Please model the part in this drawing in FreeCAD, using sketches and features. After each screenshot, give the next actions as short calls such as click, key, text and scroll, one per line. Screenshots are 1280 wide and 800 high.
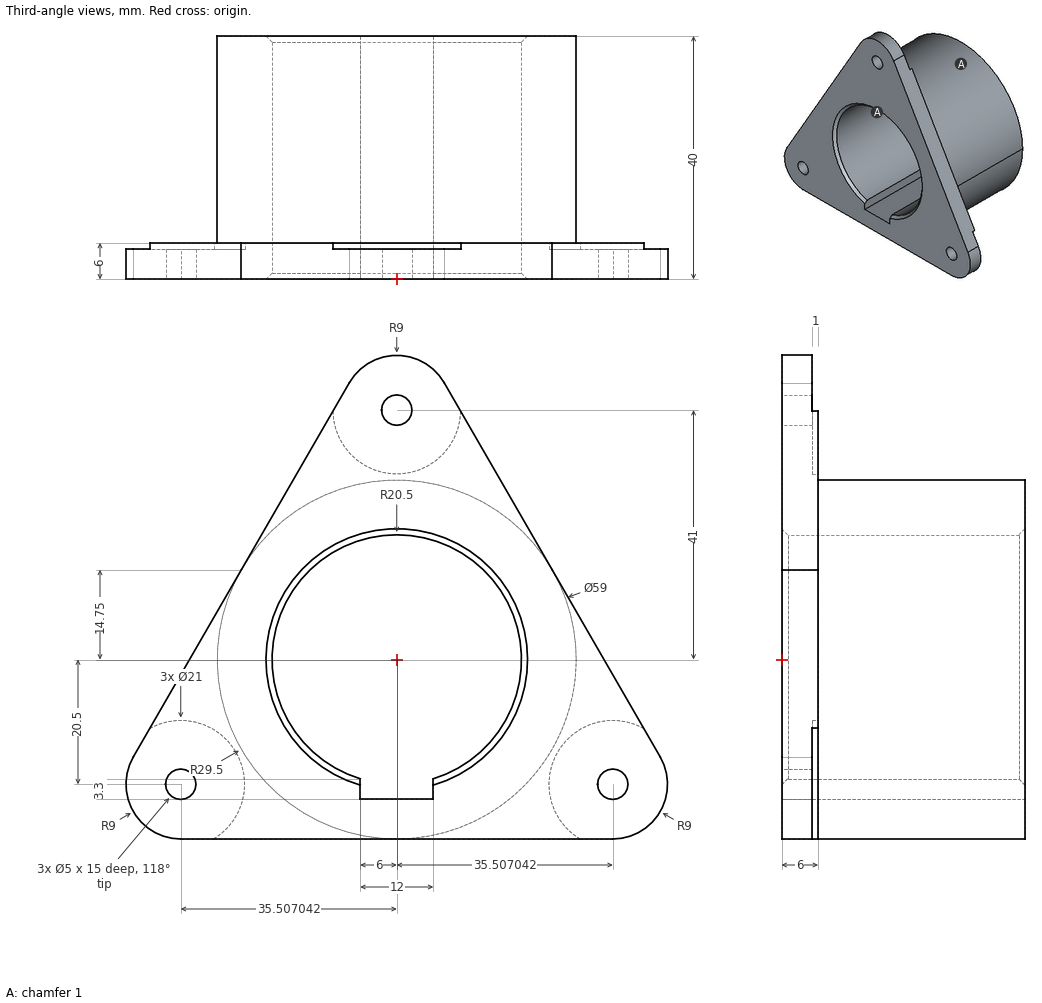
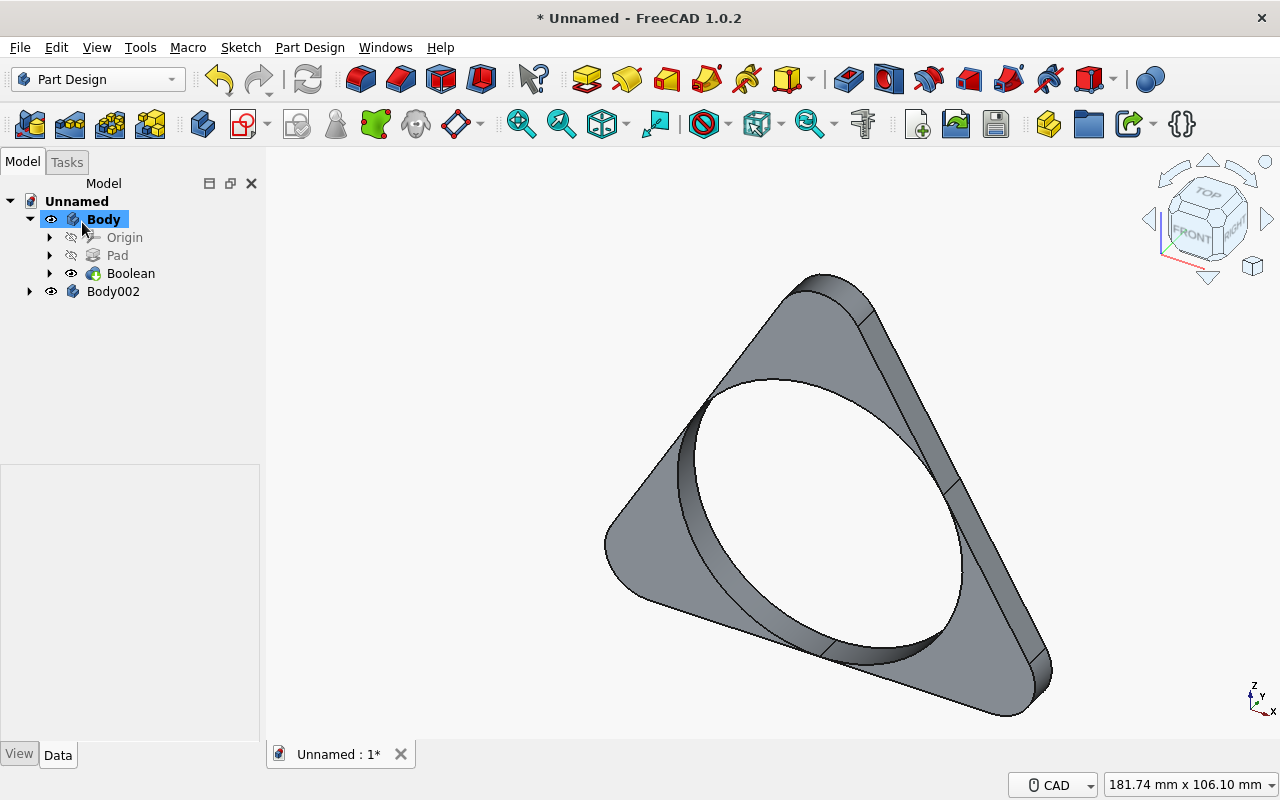
click(96, 291)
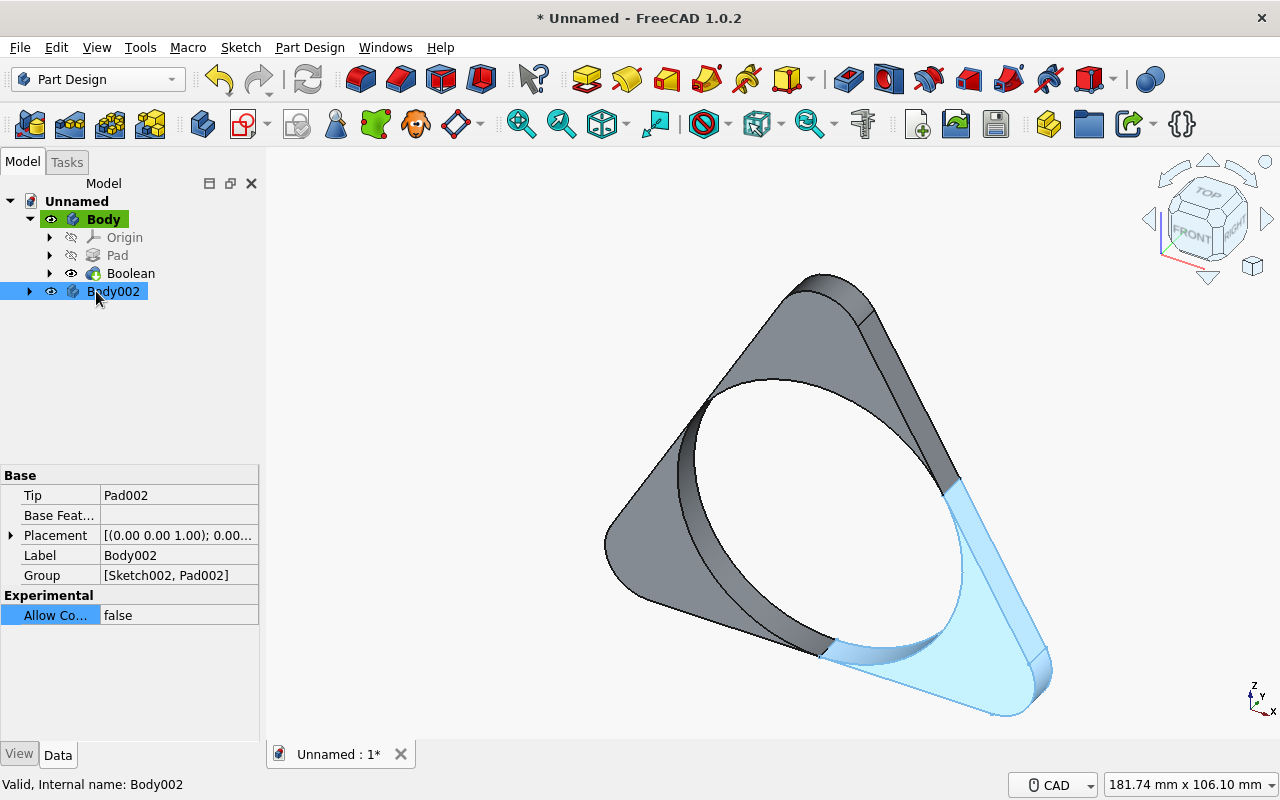
click(1152, 80)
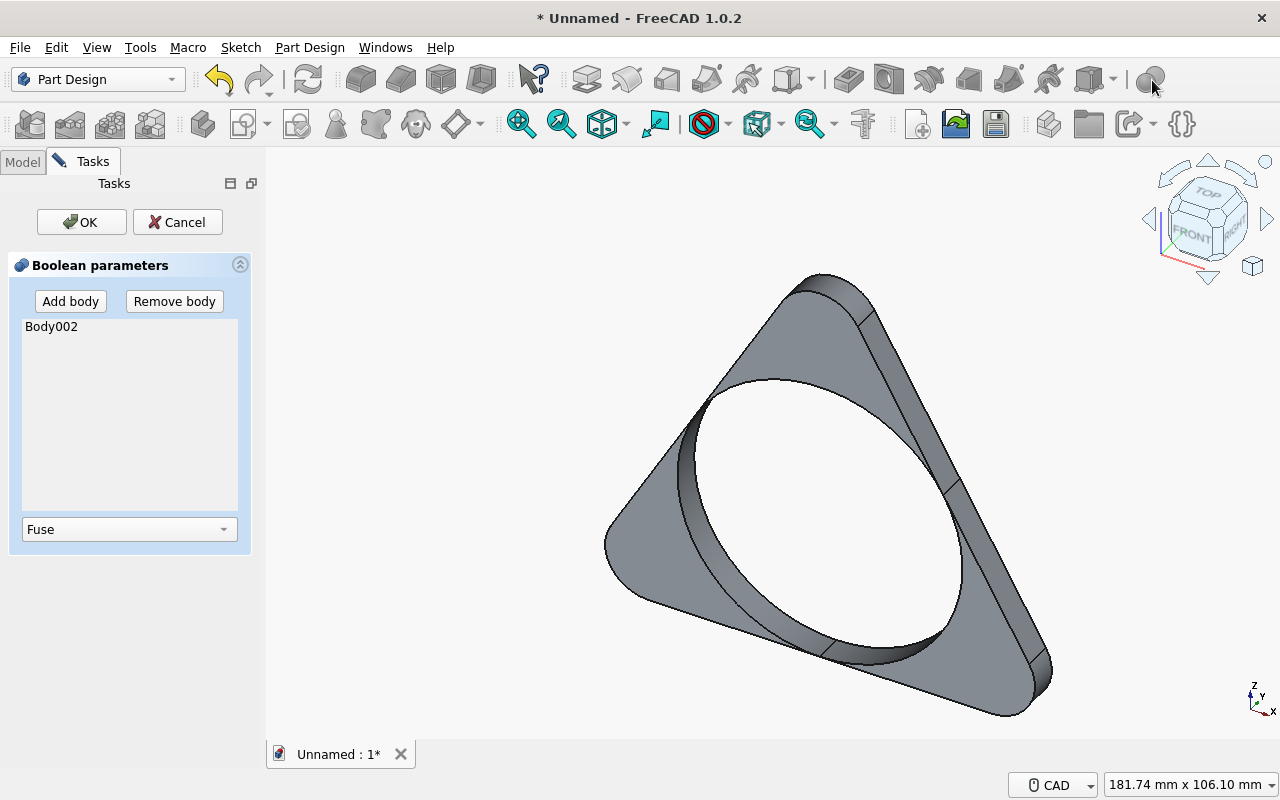
click(82, 222)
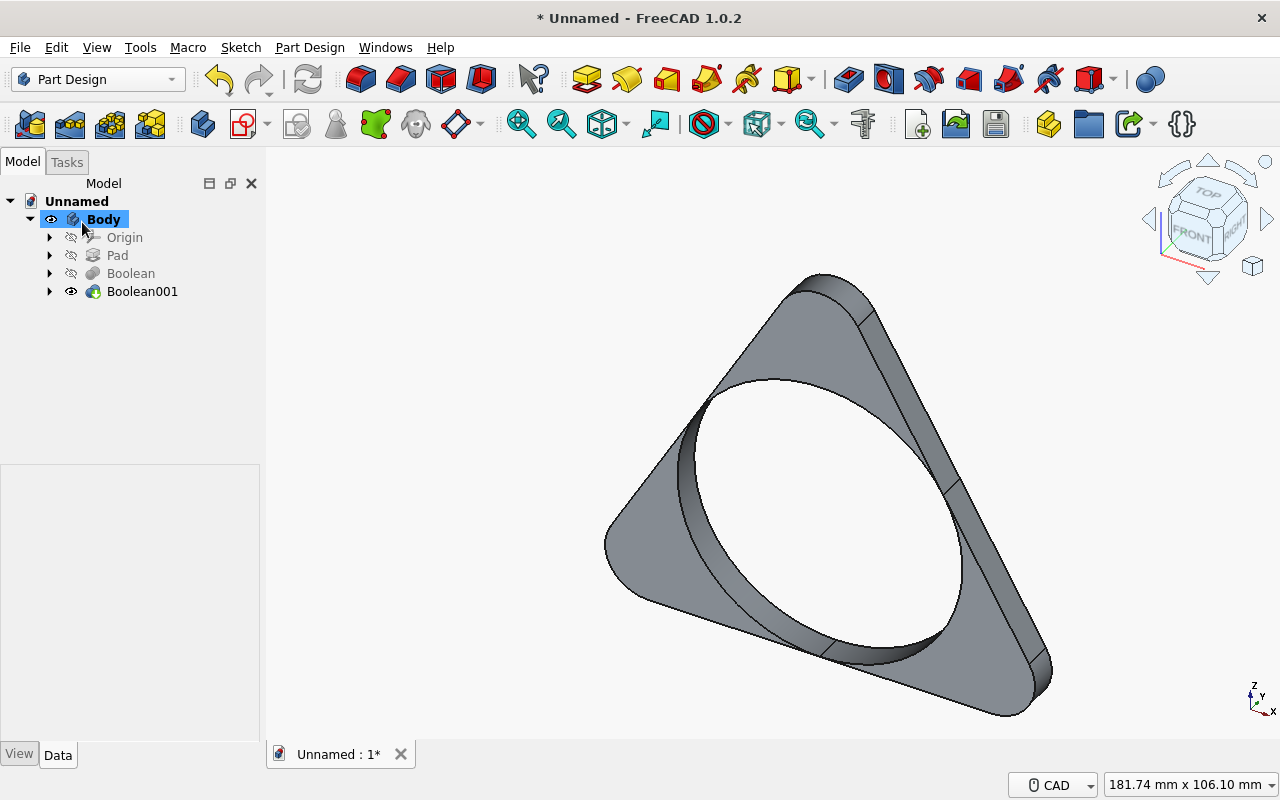
click(820, 350)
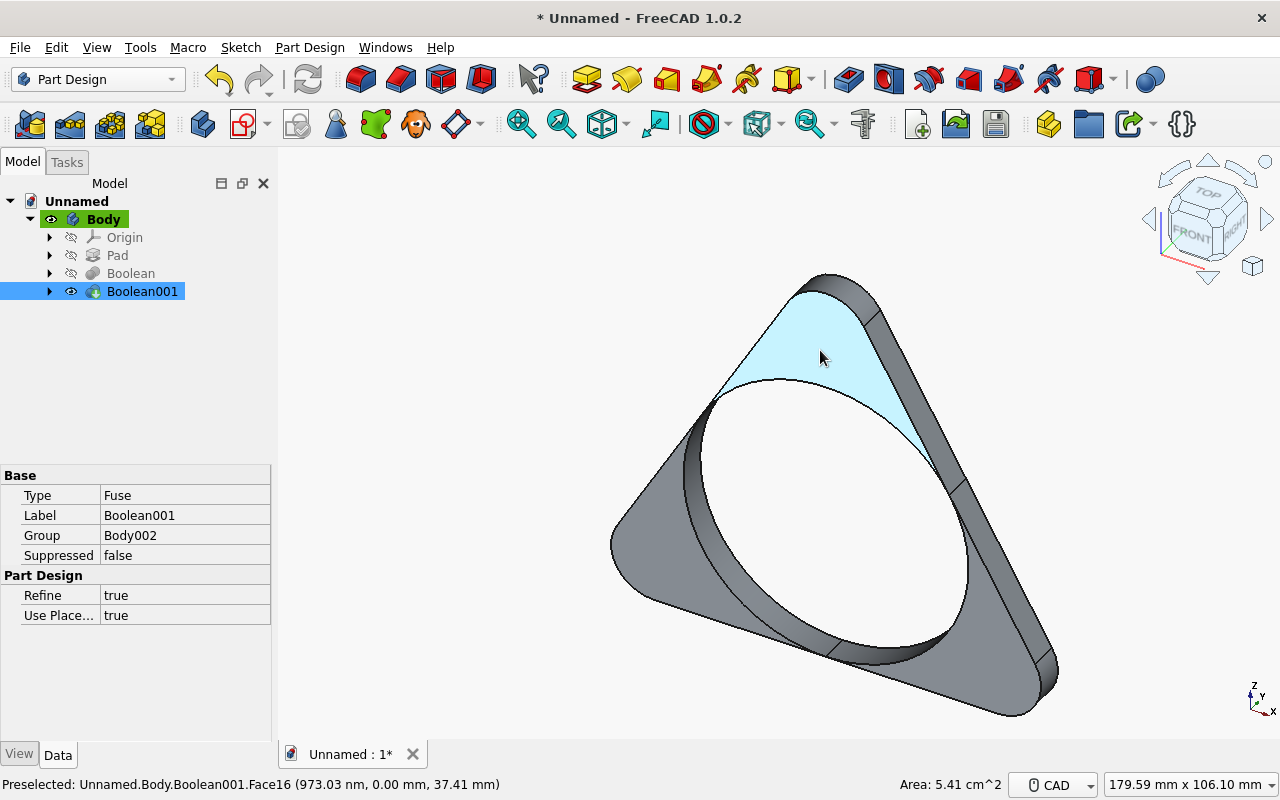
click(244, 124)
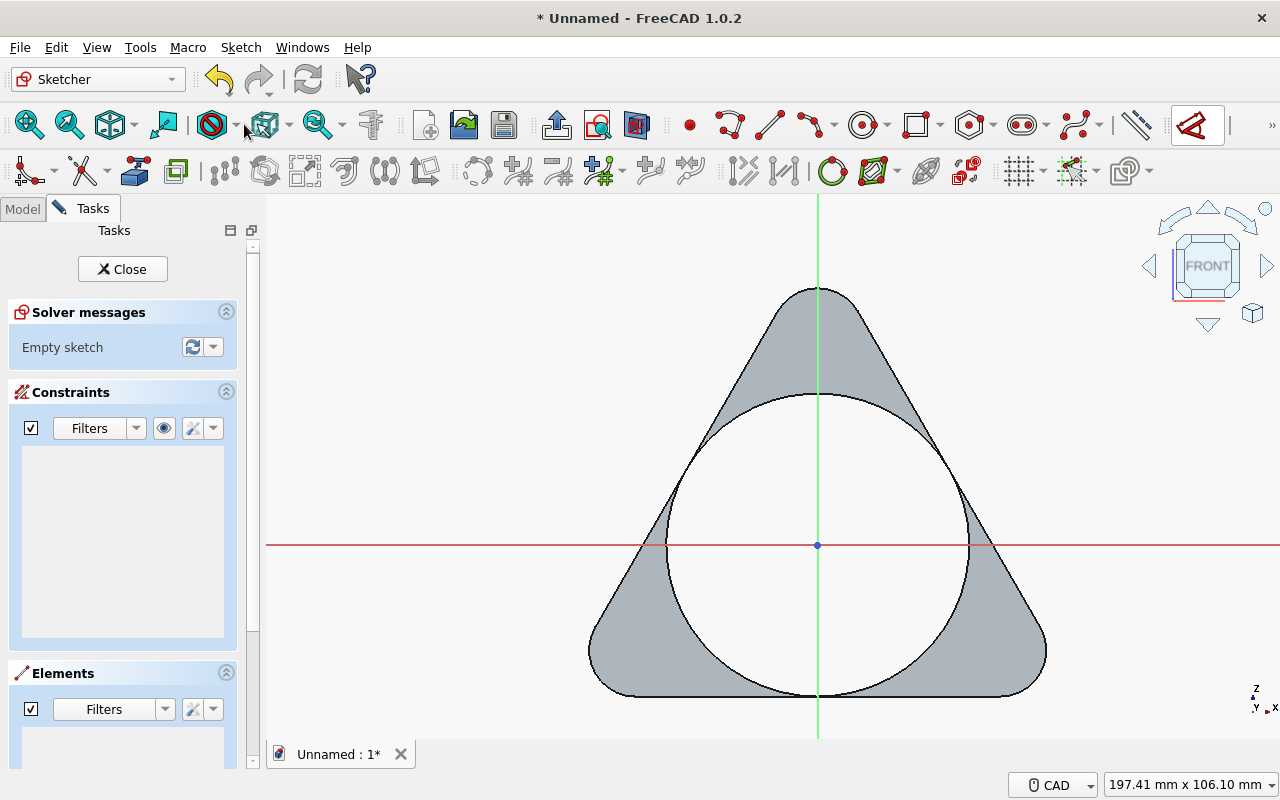
scroll(294, 222, down, 1)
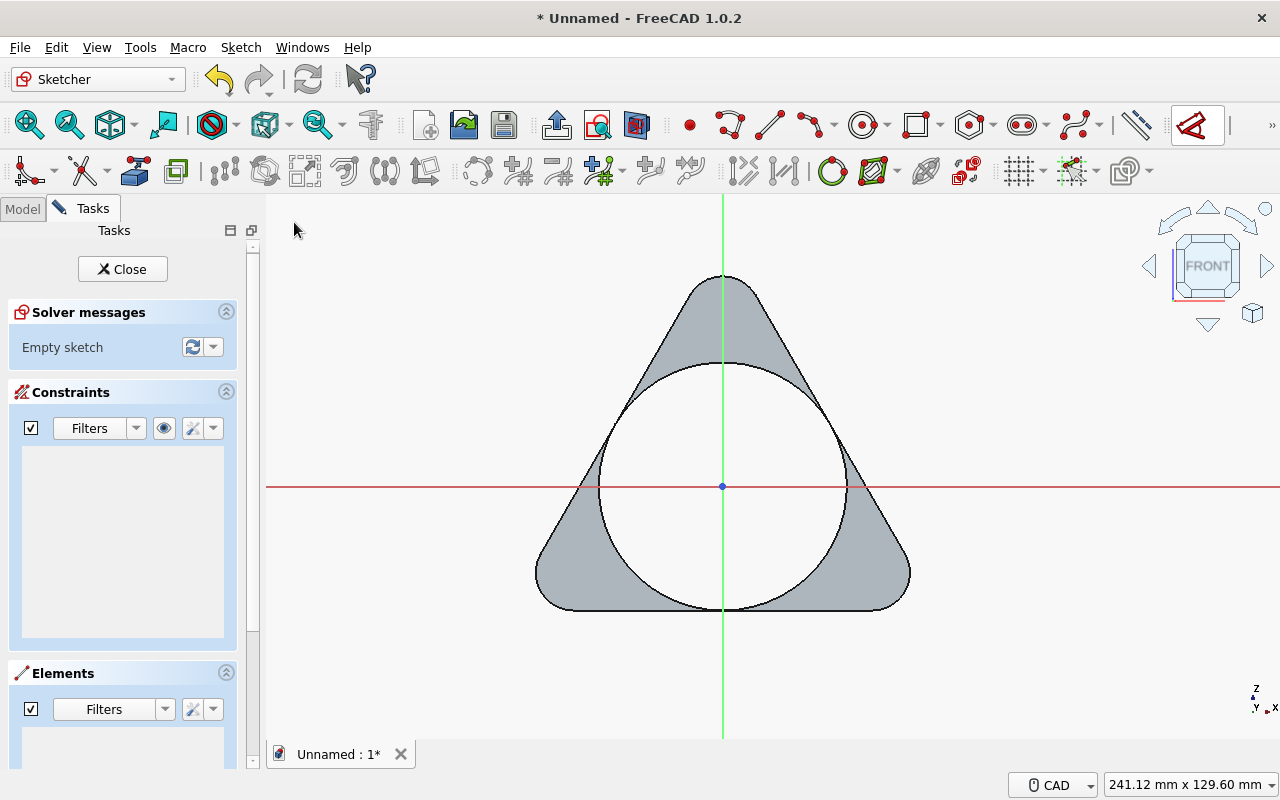
scroll(760, 527, up, 2)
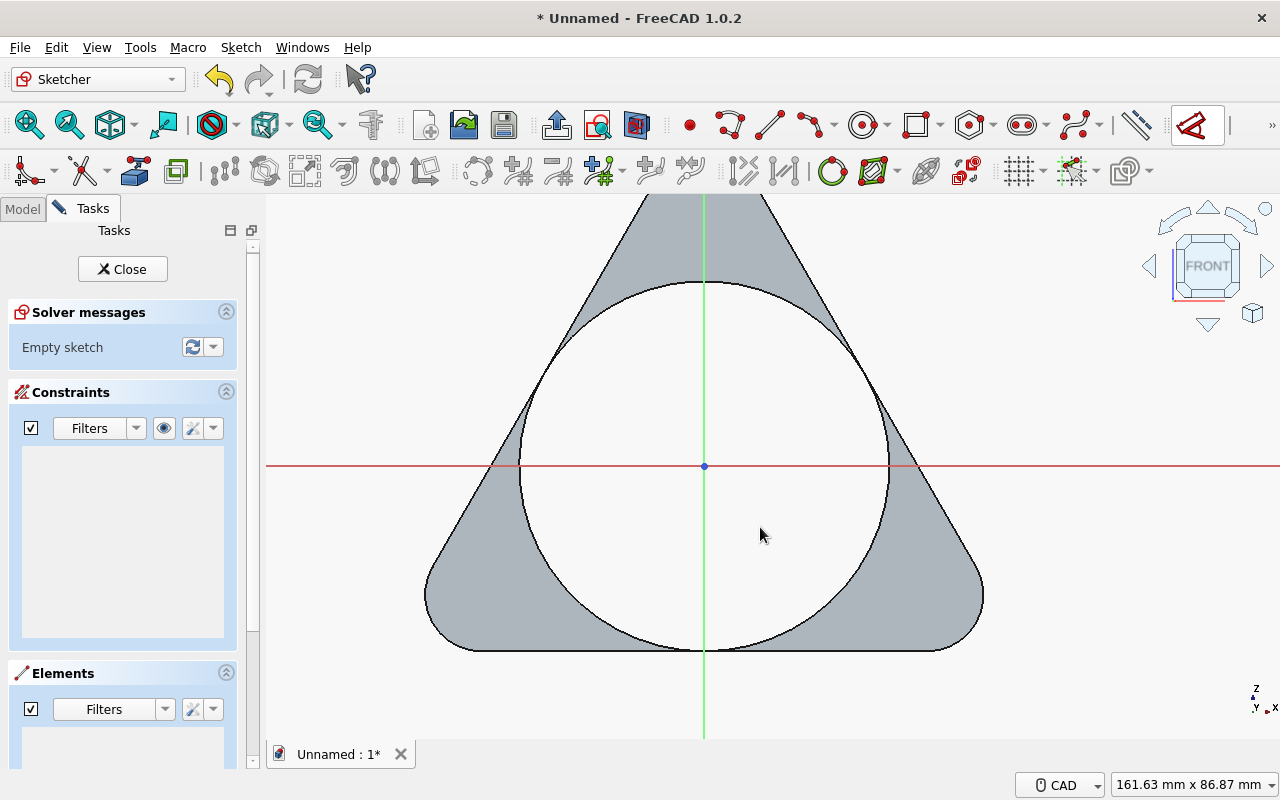
click(730, 126)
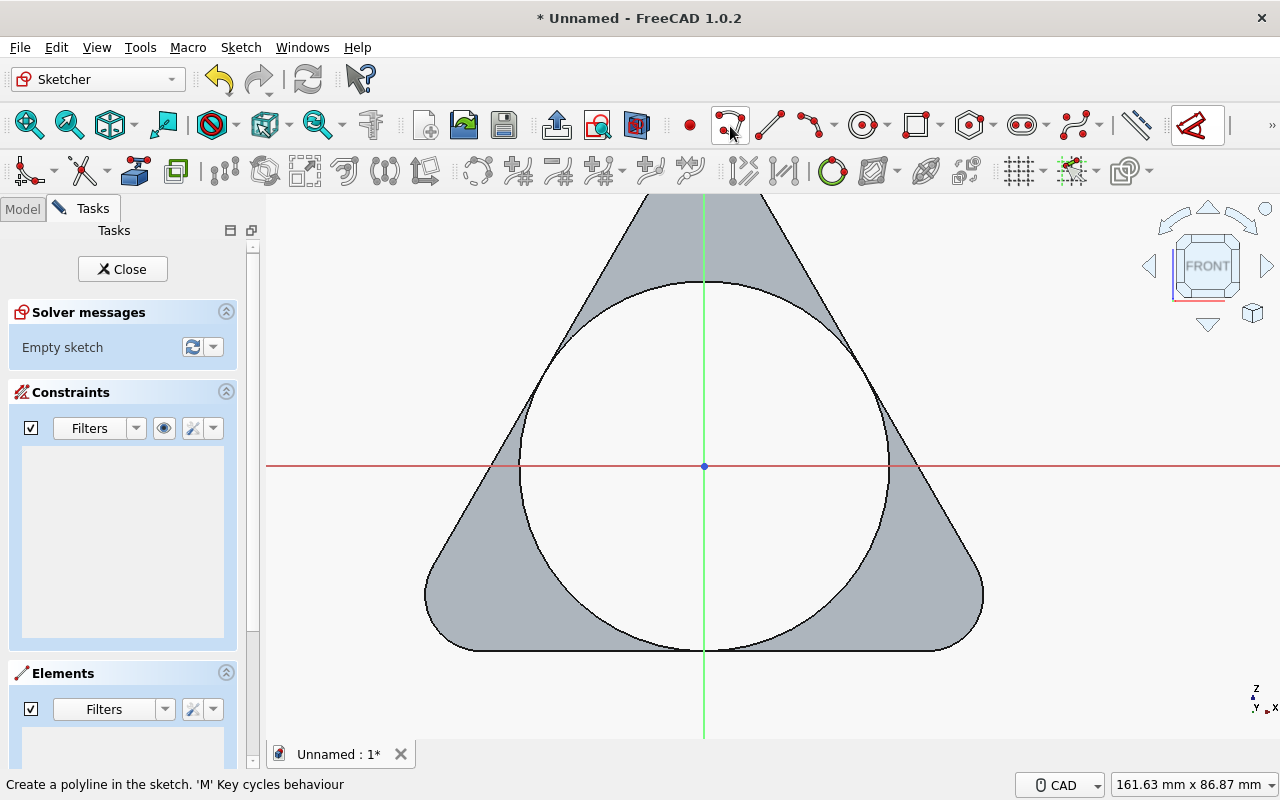
click(667, 589)
click(667, 610)
click(742, 610)
click(742, 589)
right_click(742, 589)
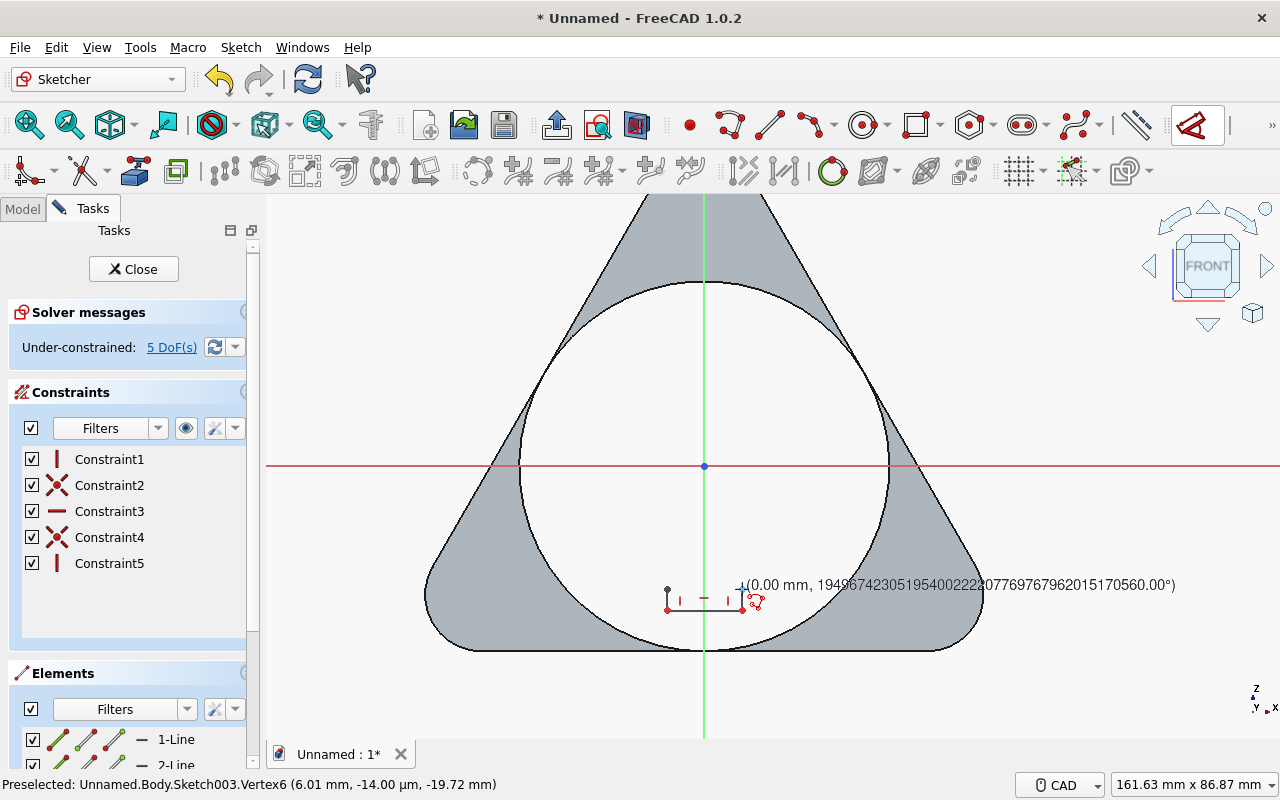
click(810, 126)